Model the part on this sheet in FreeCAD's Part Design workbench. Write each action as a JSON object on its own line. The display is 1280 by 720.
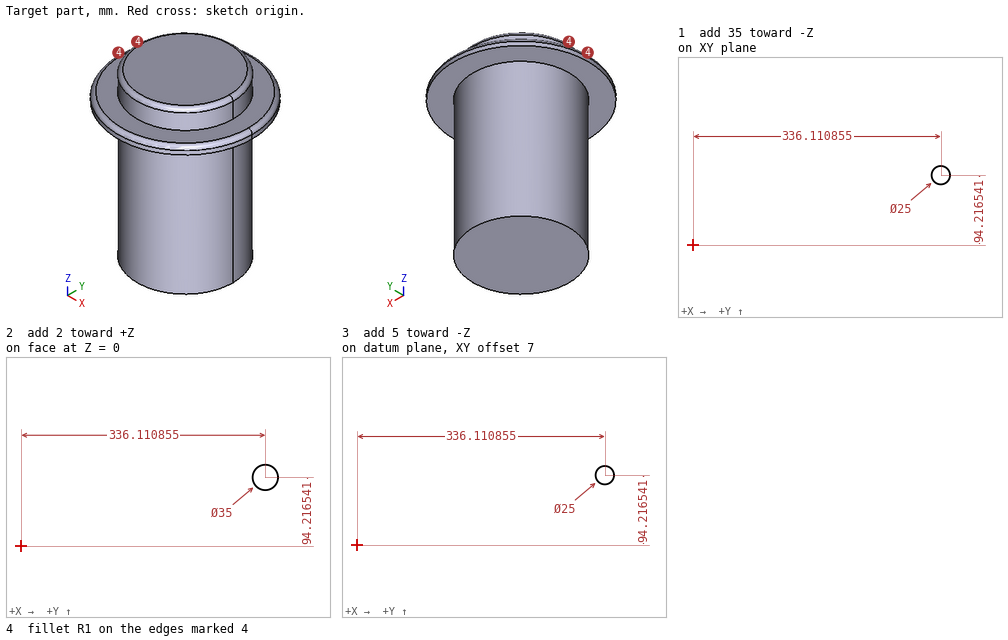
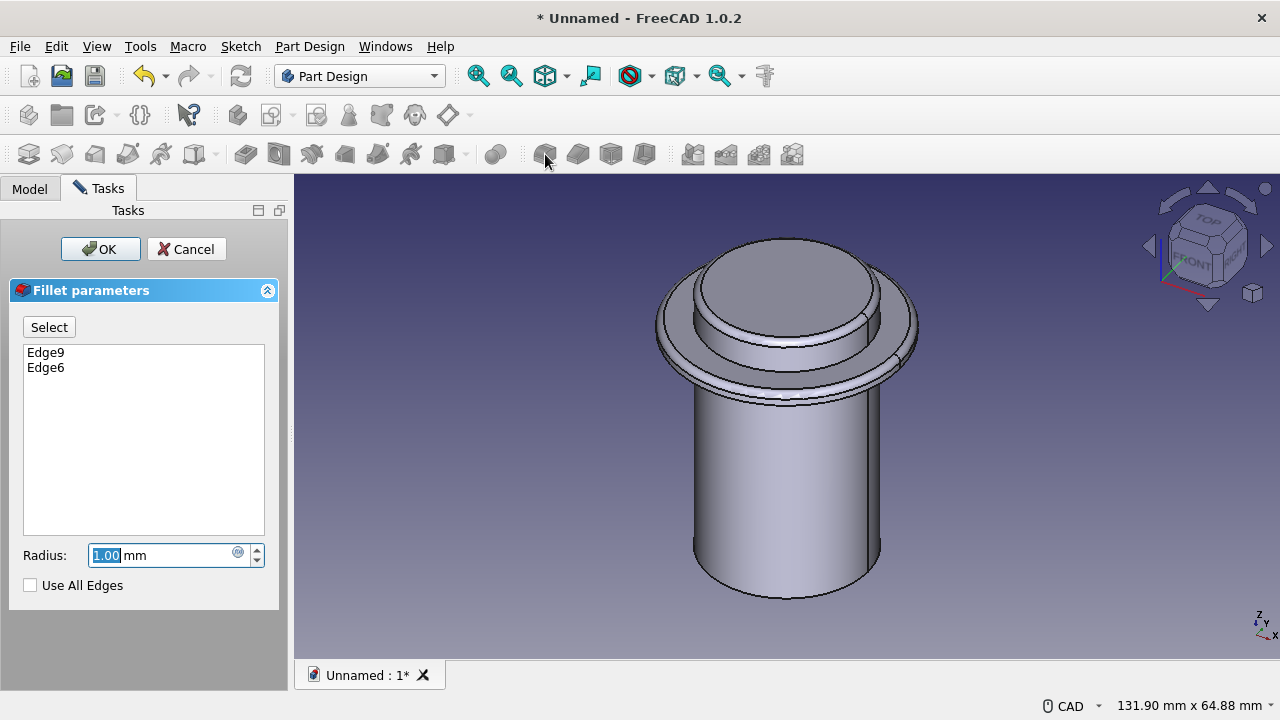
{"action": "type", "text": "1"}
{"action": "key", "text": "Tab"}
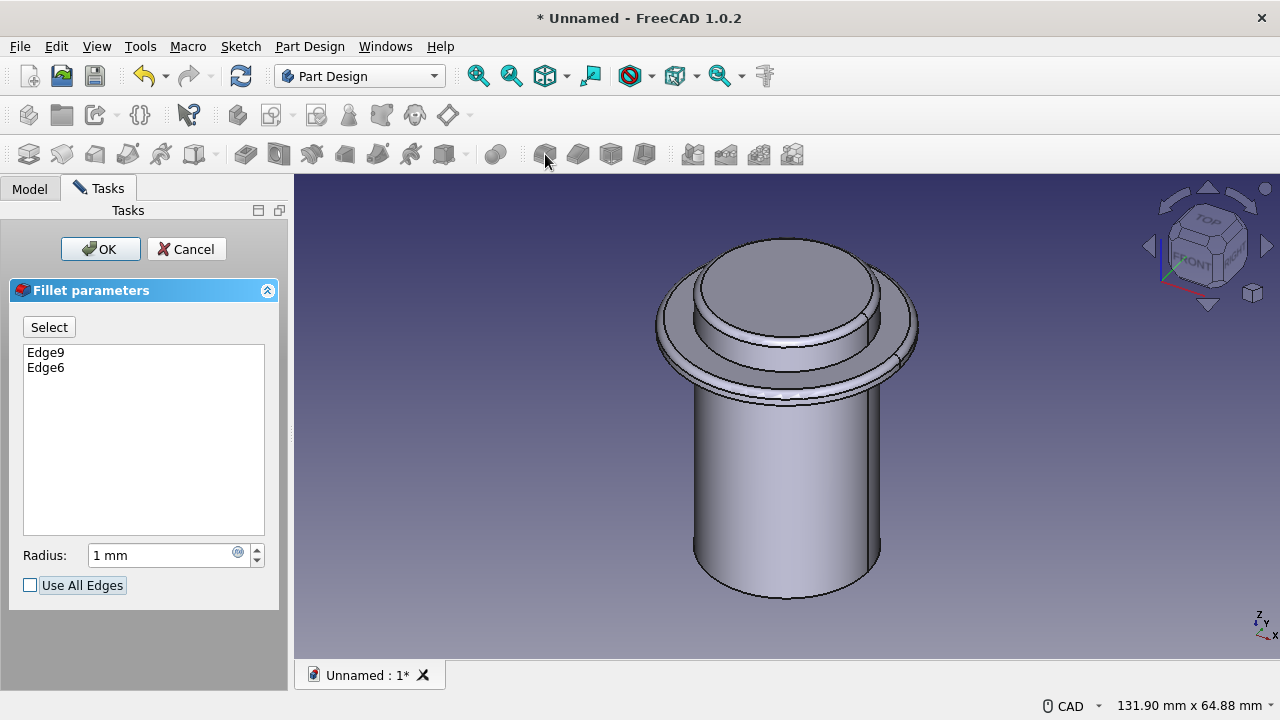
{"action": "left_click", "coordinate": [101, 249]}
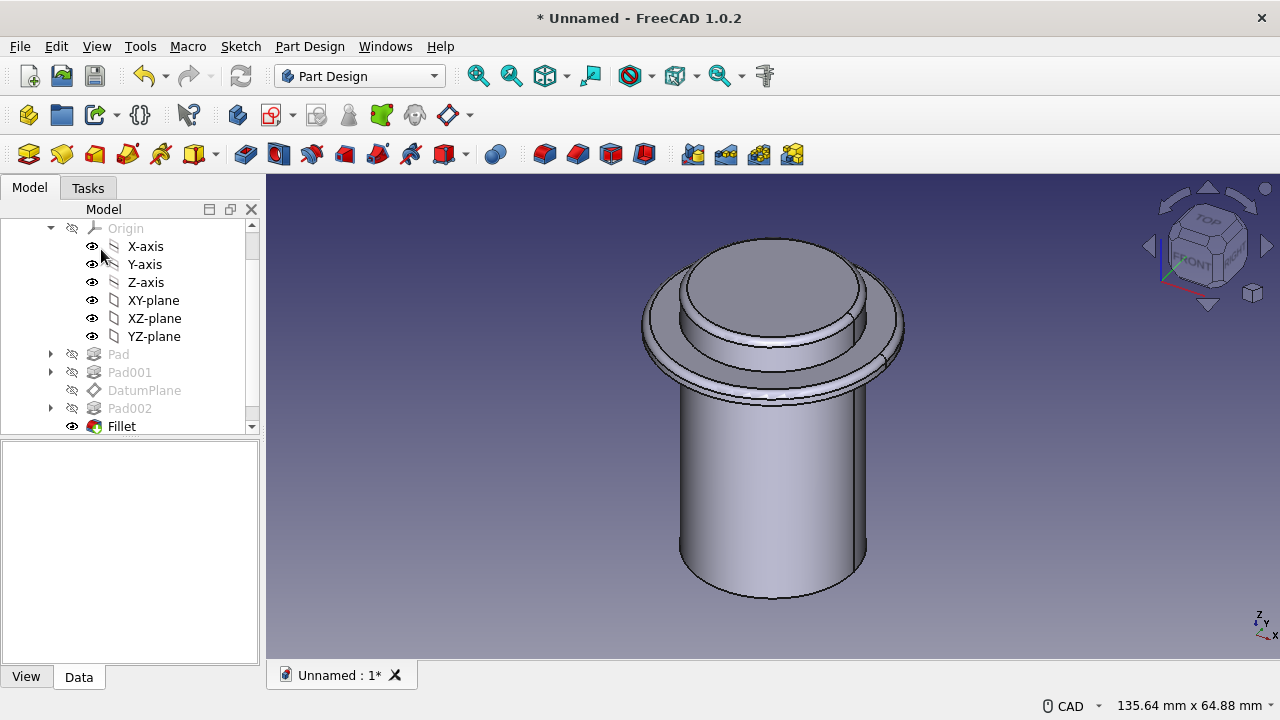
{"action": "key", "text": "0"}